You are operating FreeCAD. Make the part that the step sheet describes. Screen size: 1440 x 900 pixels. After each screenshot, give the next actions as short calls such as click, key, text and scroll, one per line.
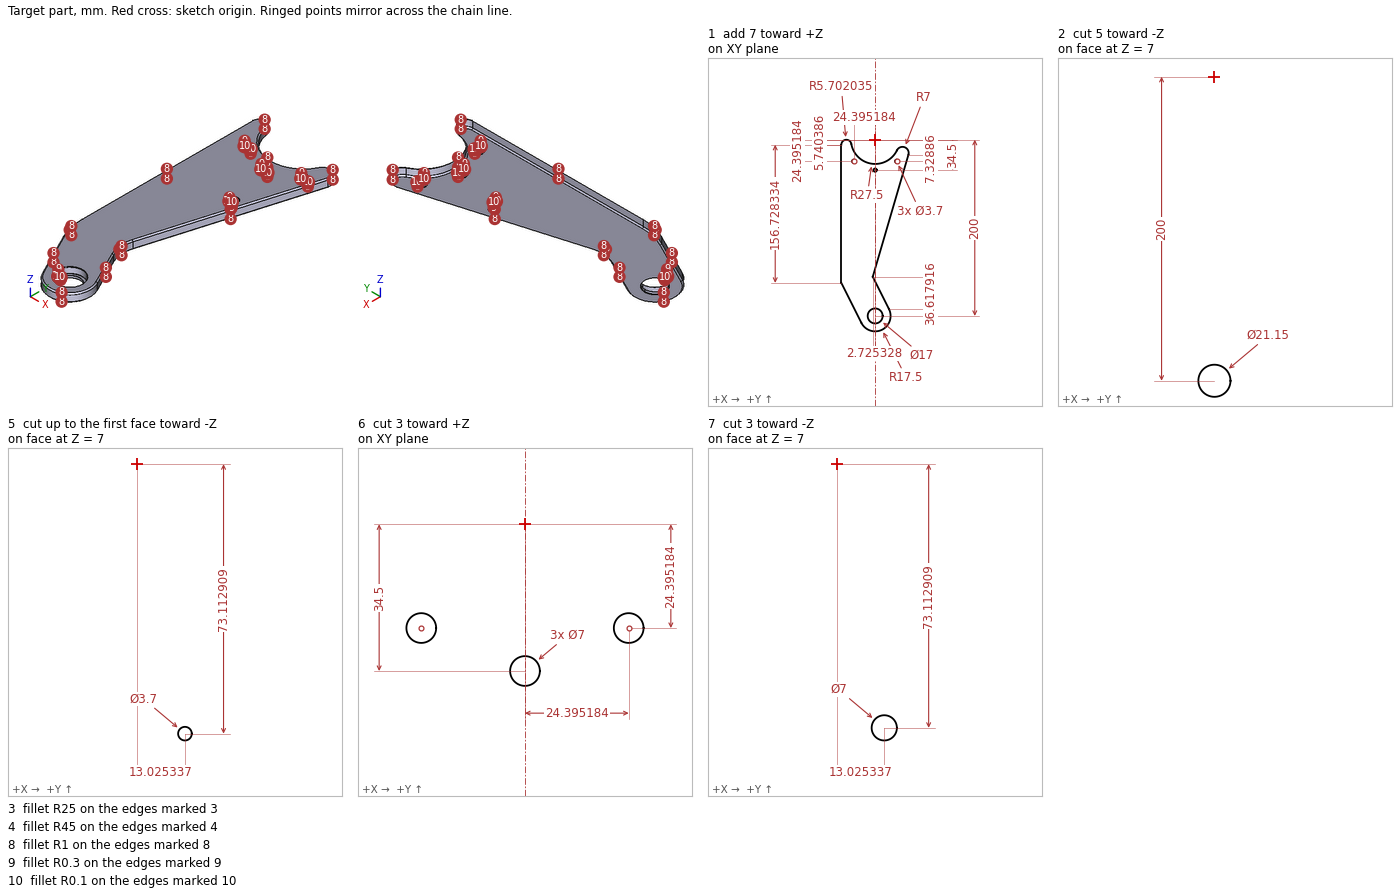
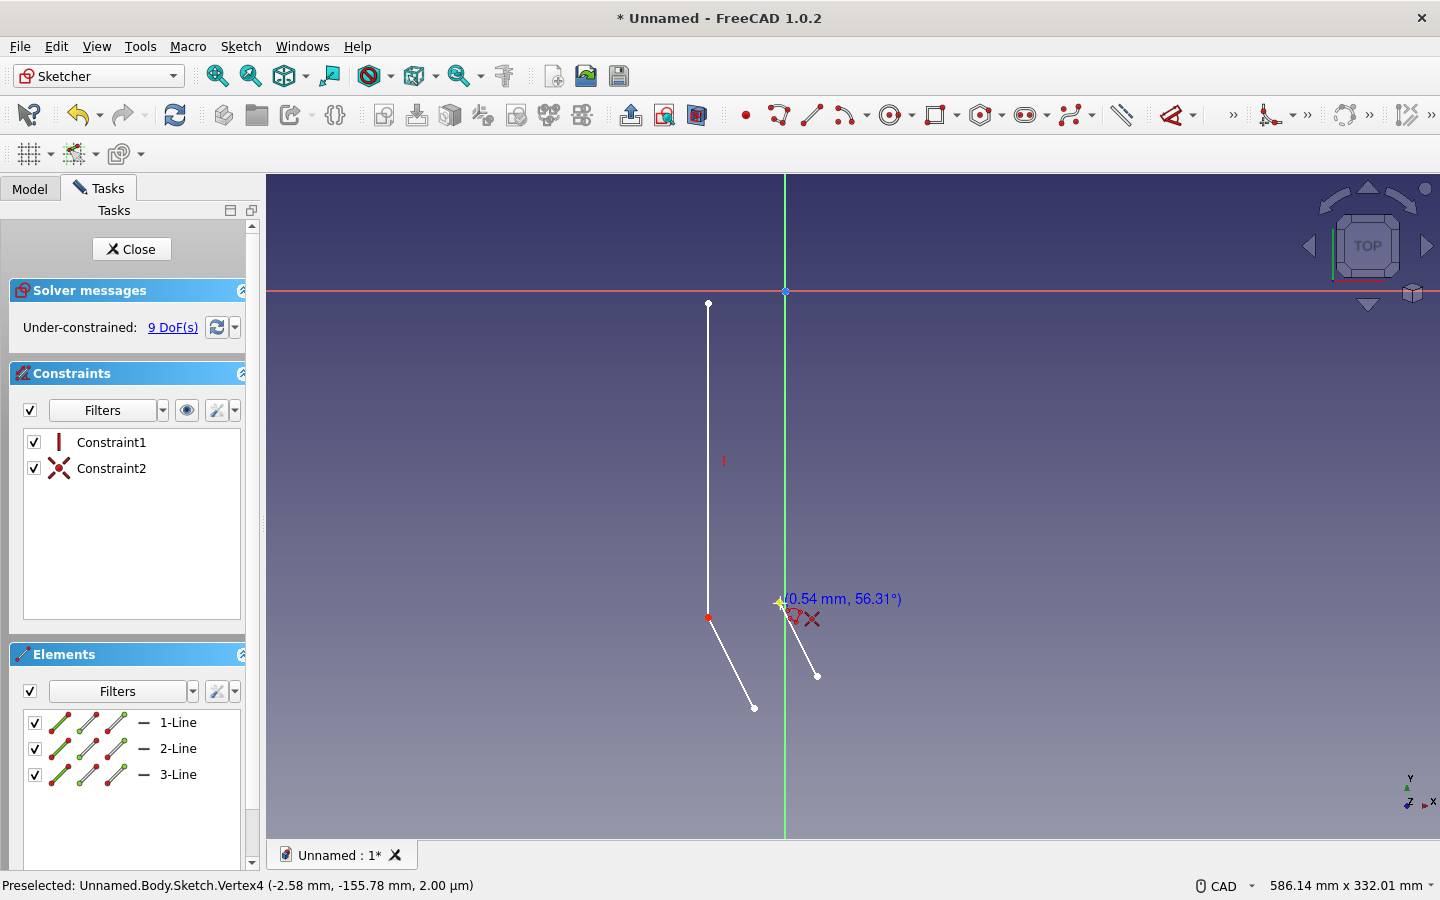
click(861, 325)
right_click(861, 325)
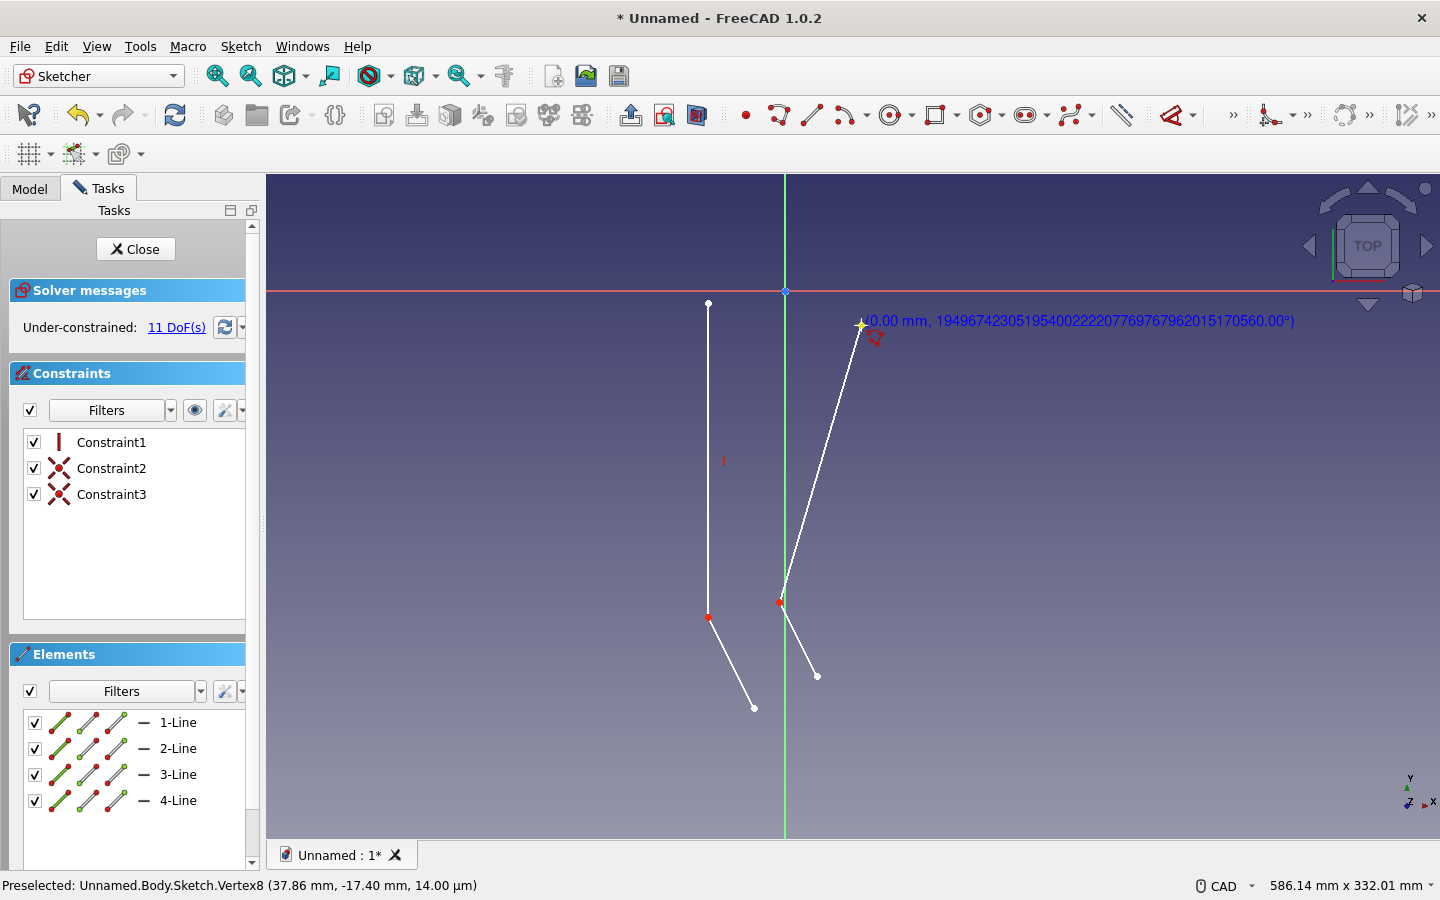
key(g)
key(3)
key(a)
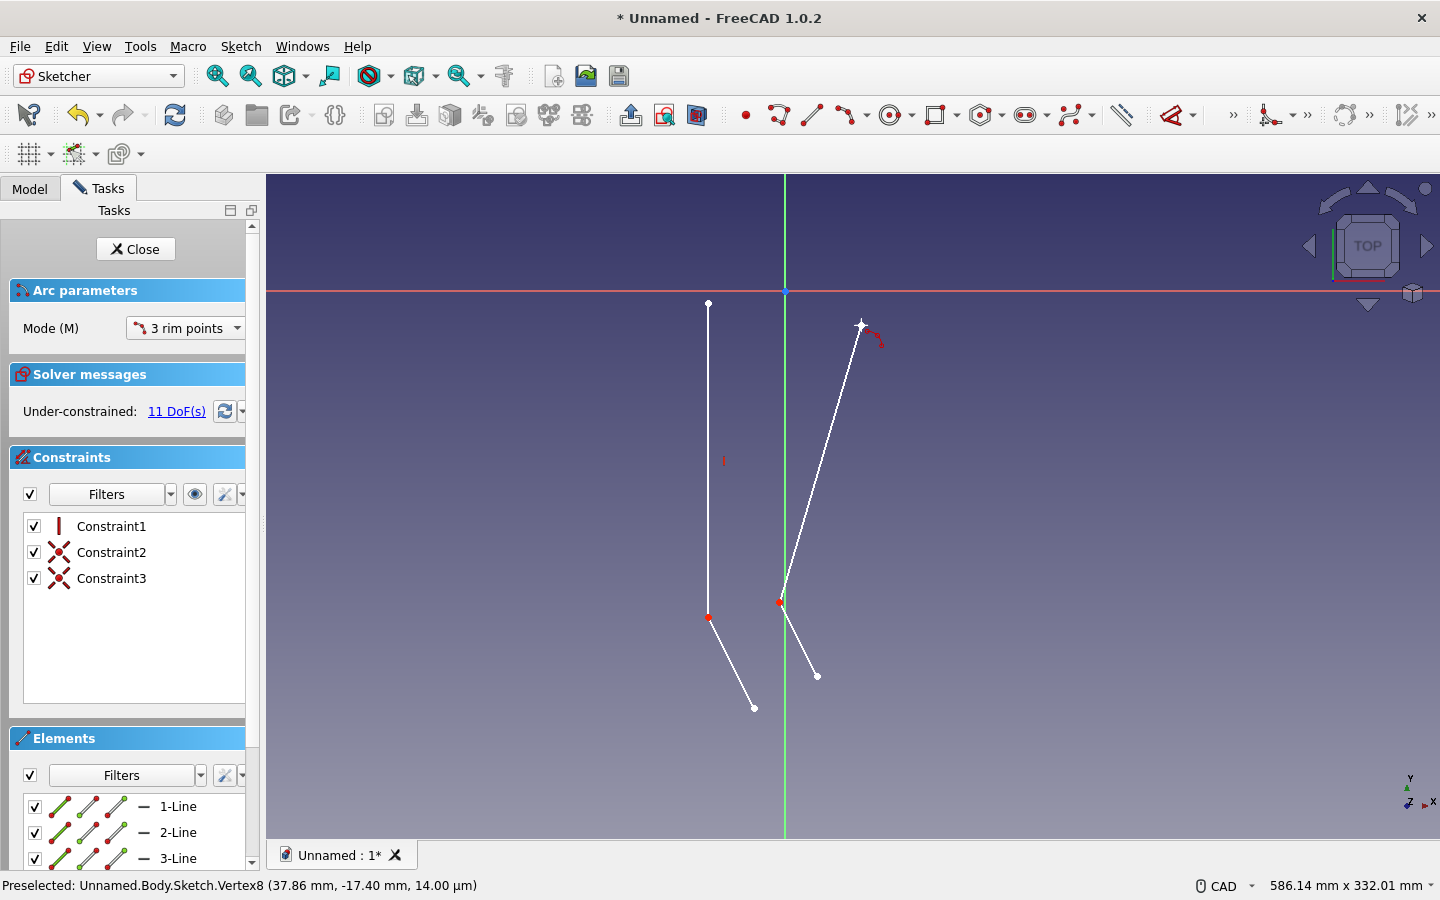
click(754, 709)
click(817, 677)
click(801, 723)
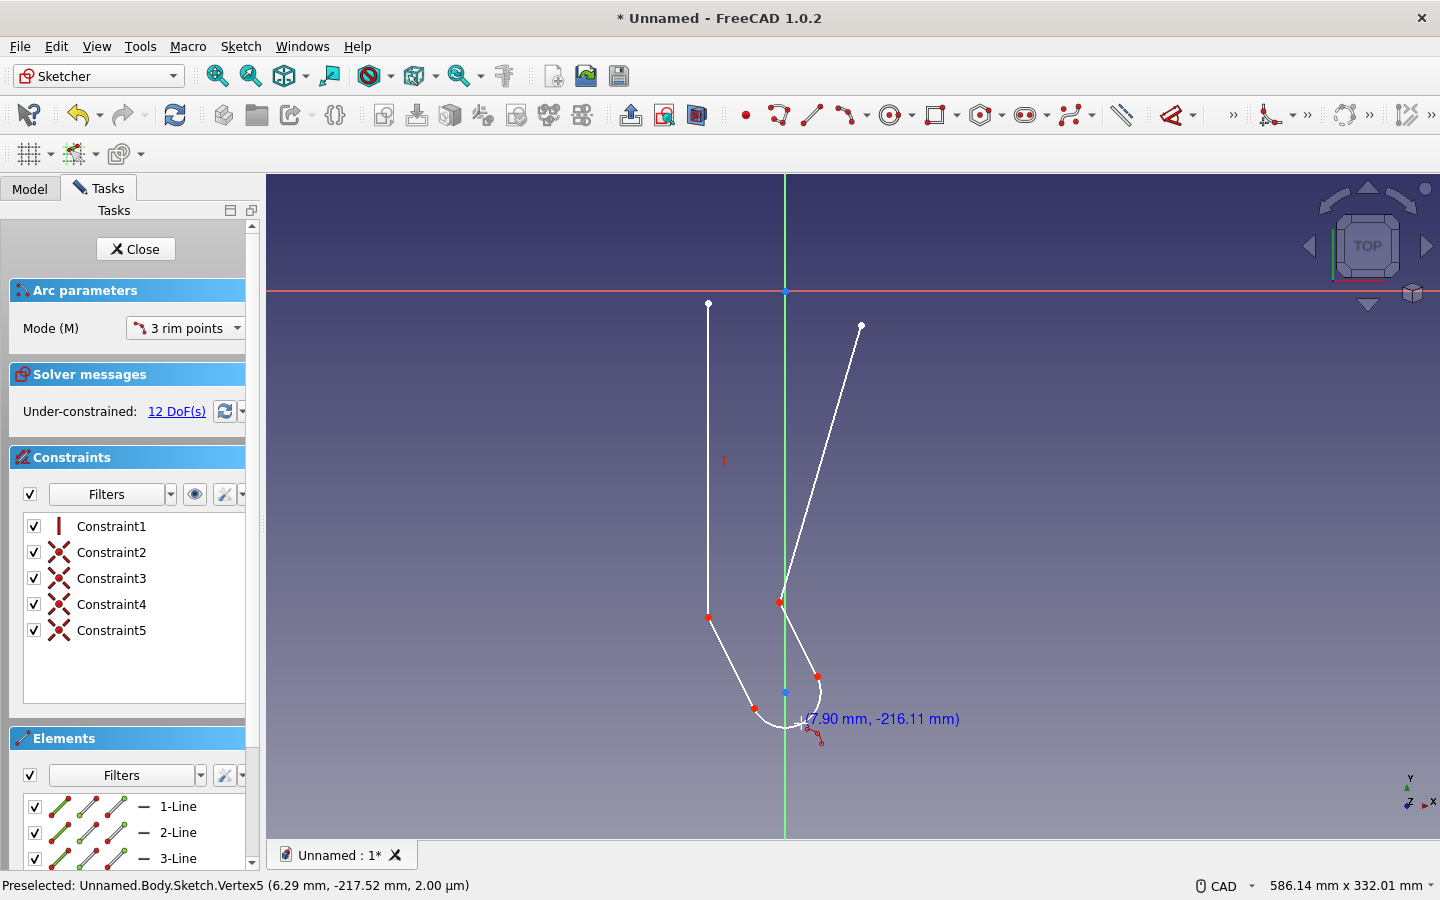
click(861, 326)
click(835, 315)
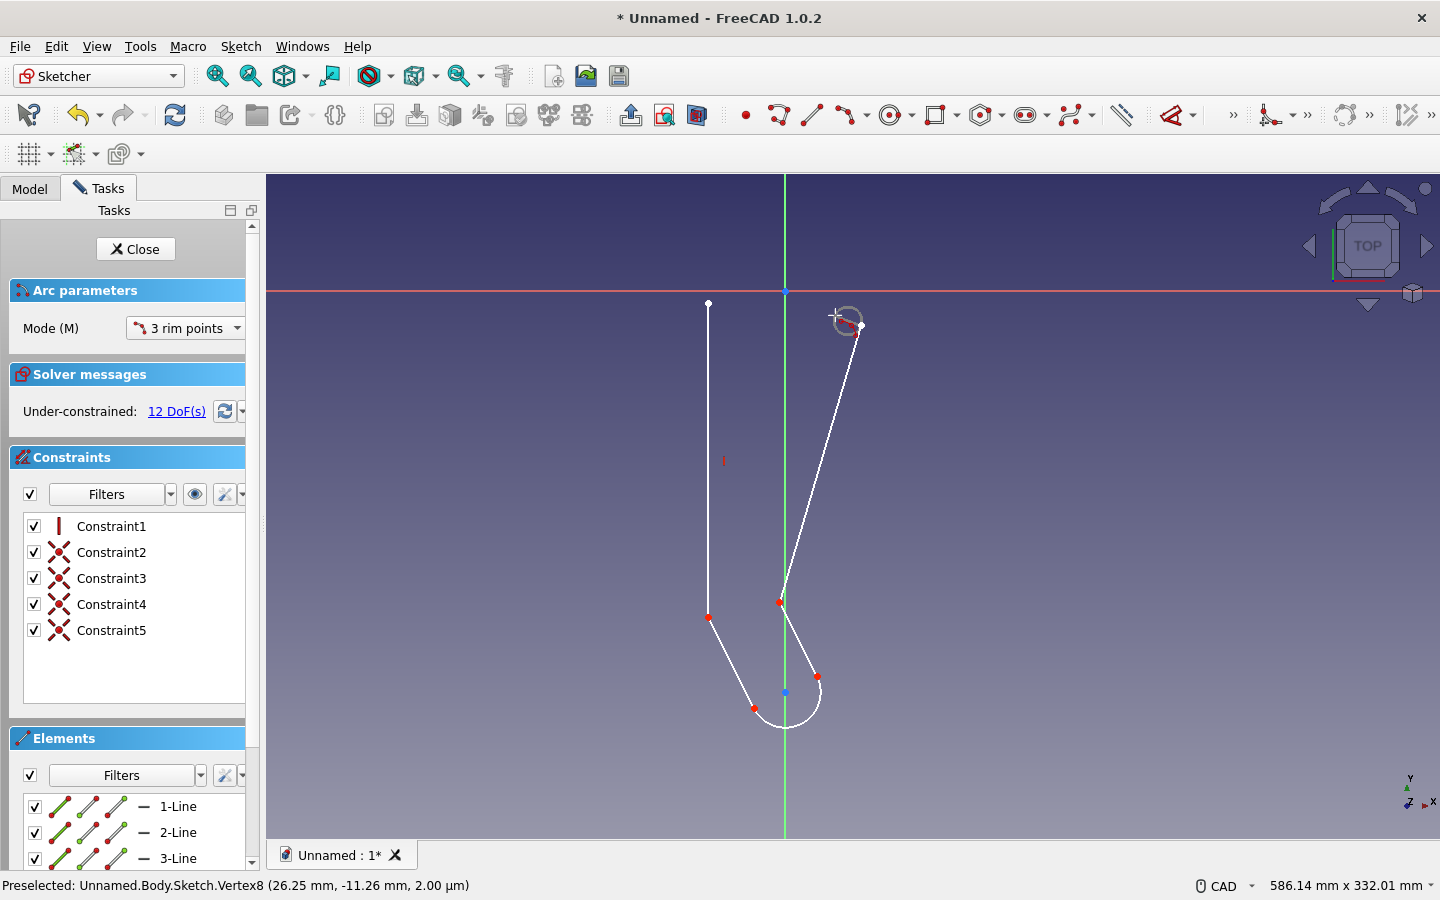
scroll(852, 308, up, 2)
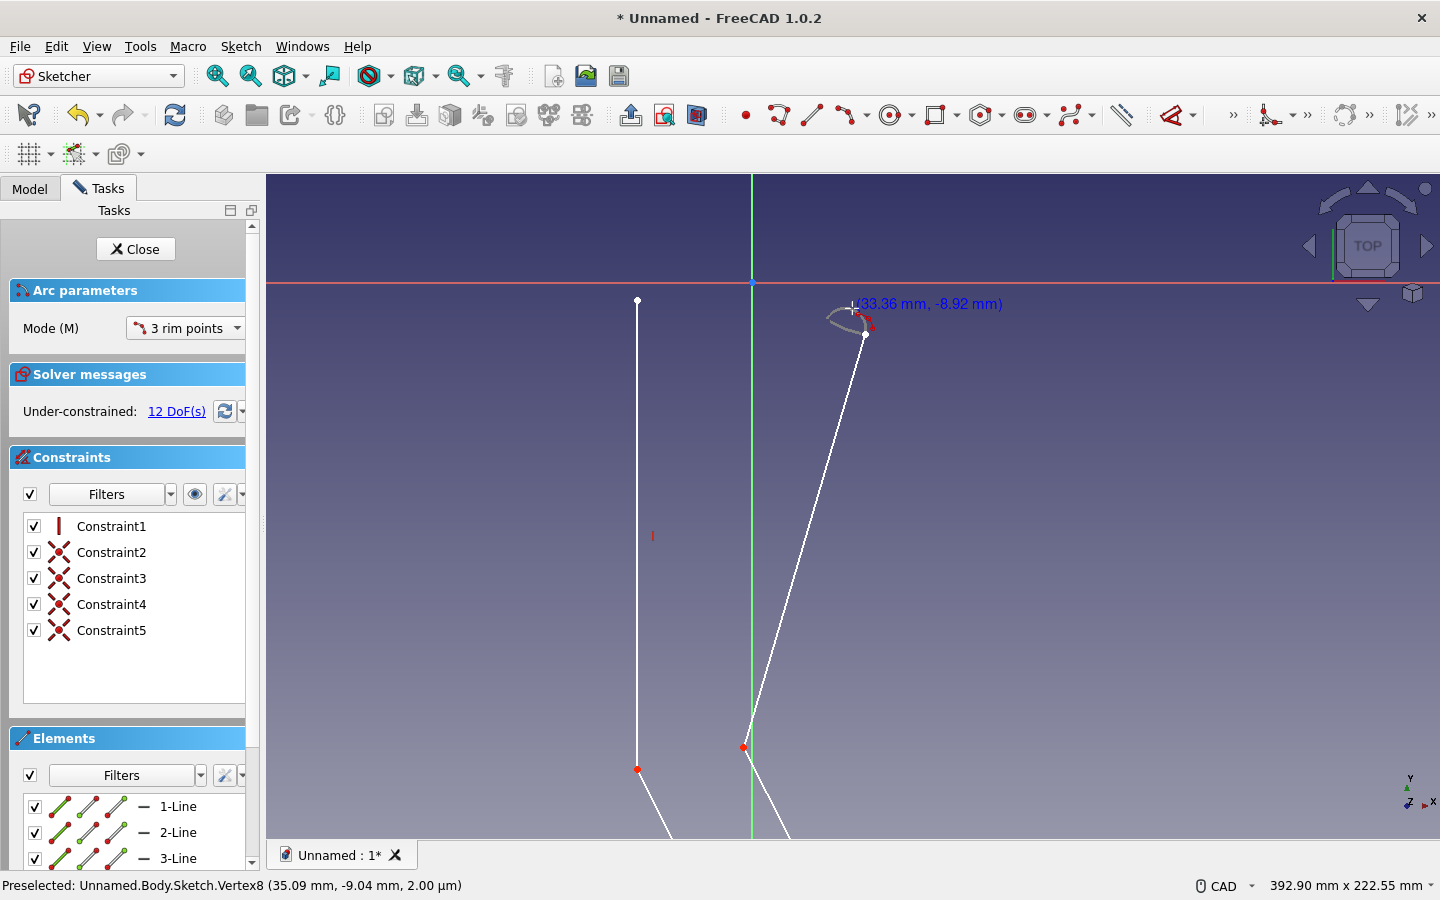
click(852, 308)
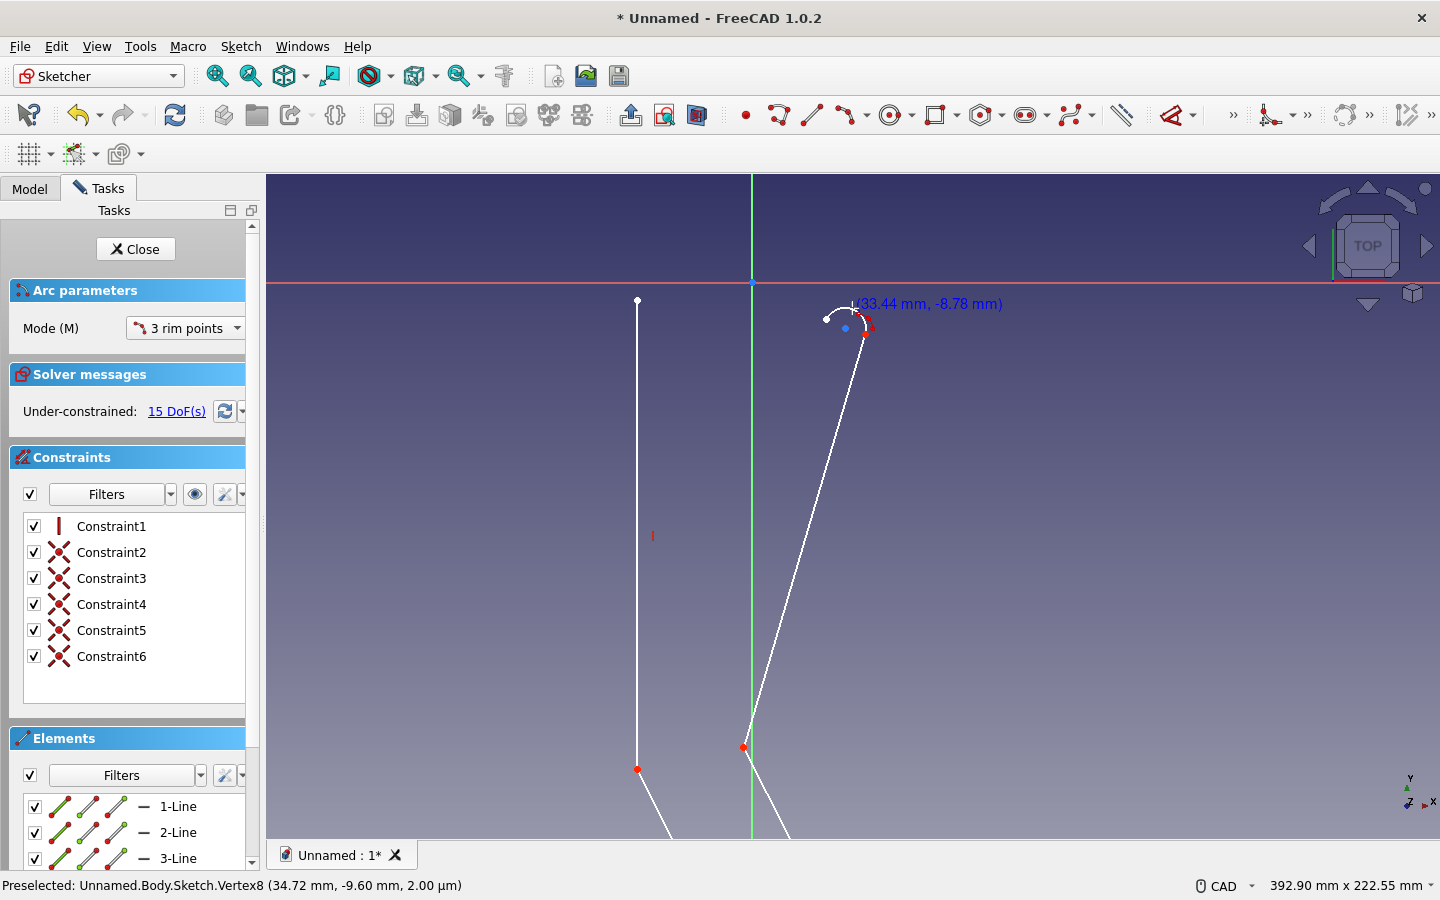
click(826, 320)
click(671, 297)
click(721, 359)